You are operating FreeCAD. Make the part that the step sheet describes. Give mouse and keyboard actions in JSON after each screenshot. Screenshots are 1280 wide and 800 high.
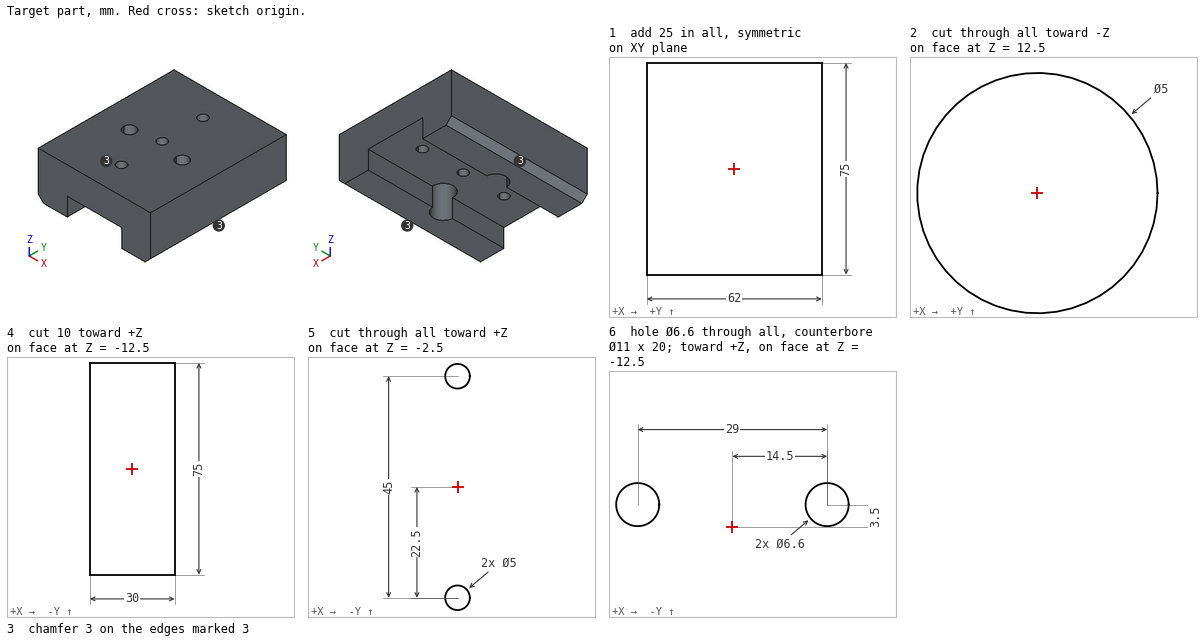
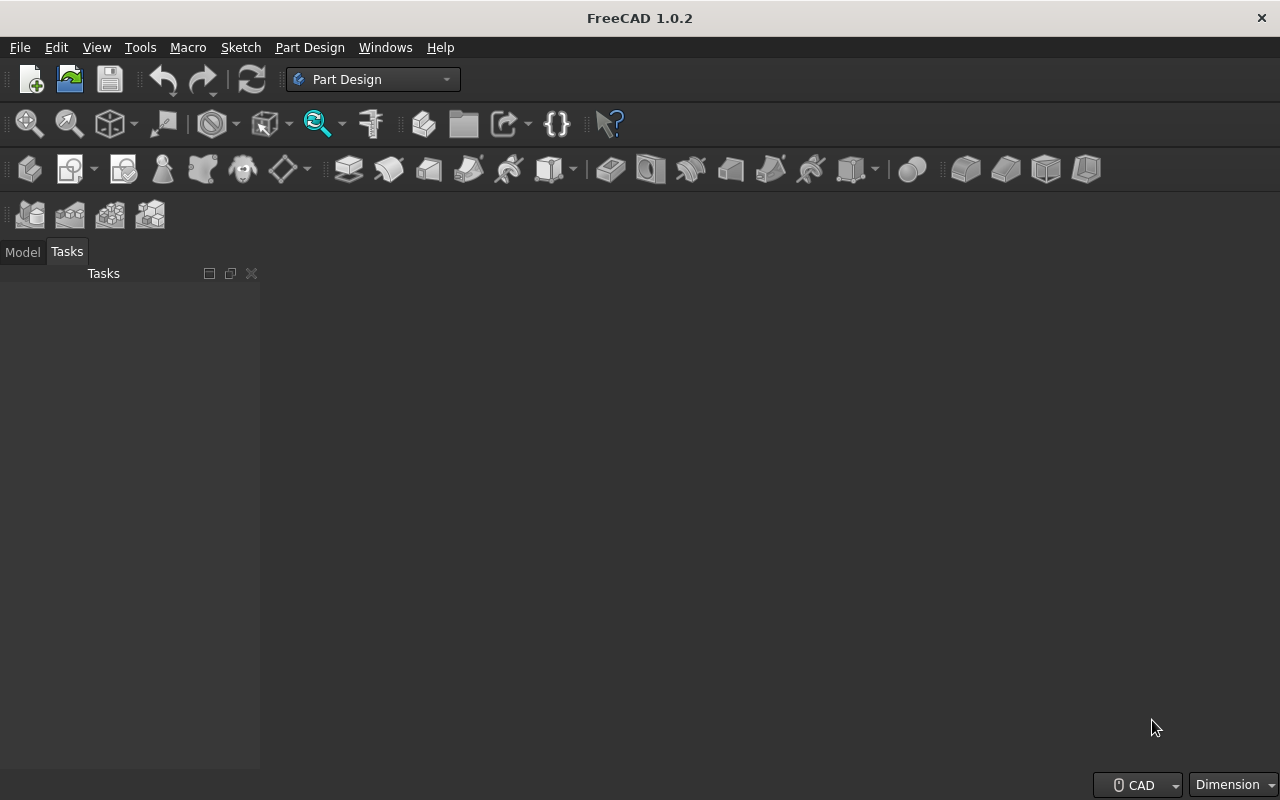
{"action": "left_click", "coordinate": [30, 80]}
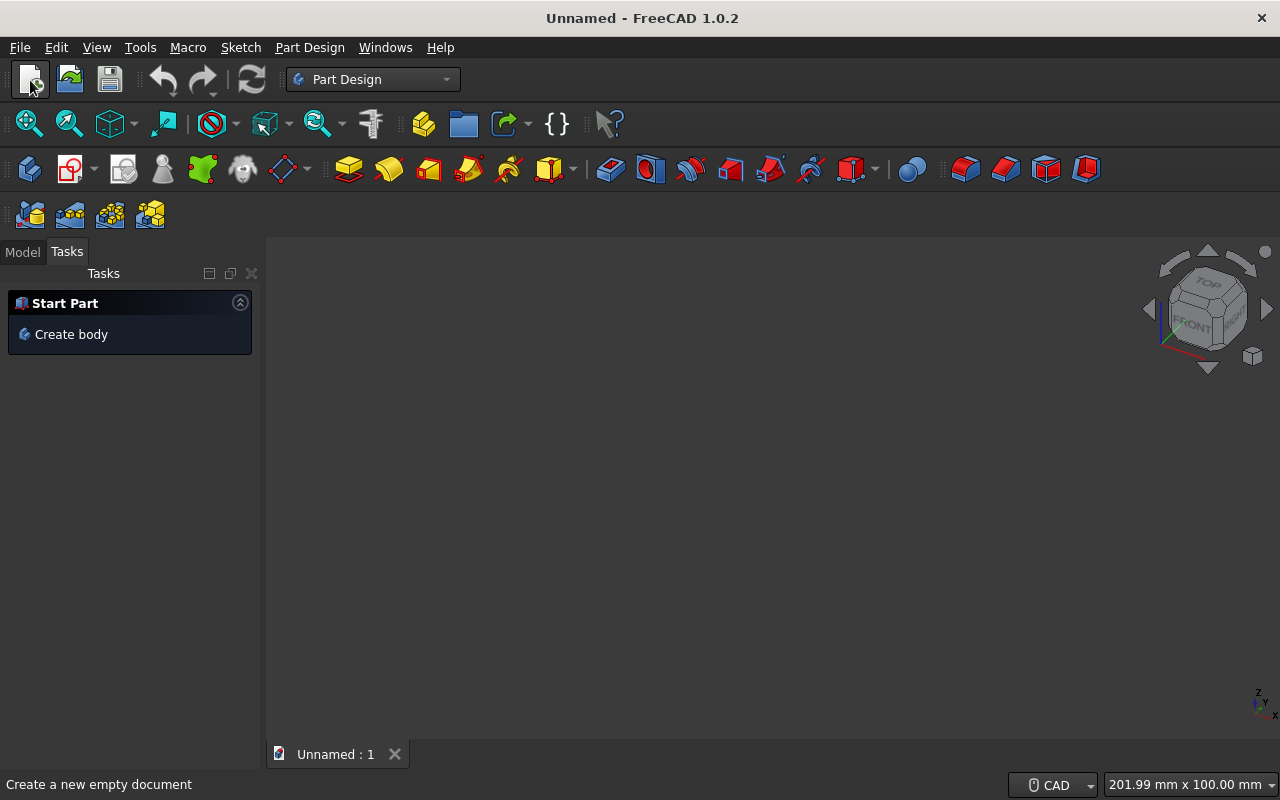
{"action": "left_click", "coordinate": [70, 170]}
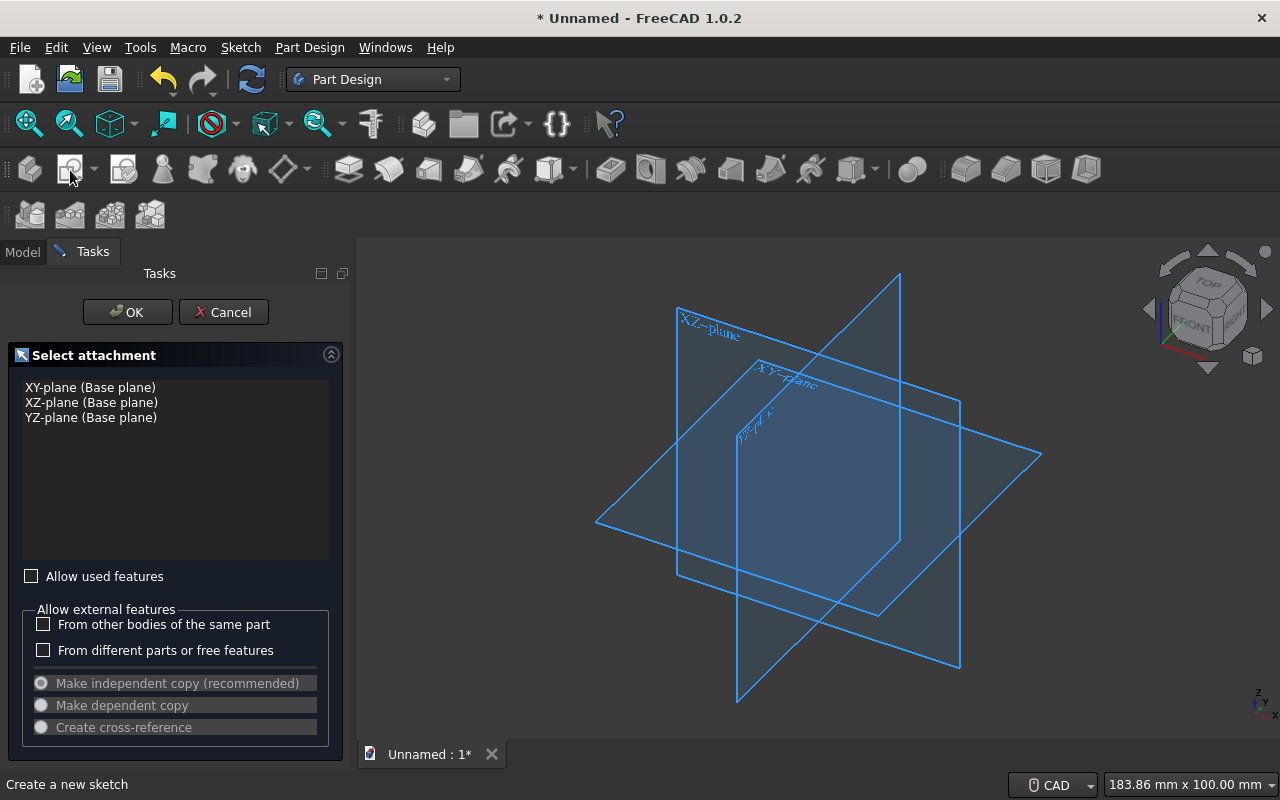
{"action": "left_click", "coordinate": [82, 388]}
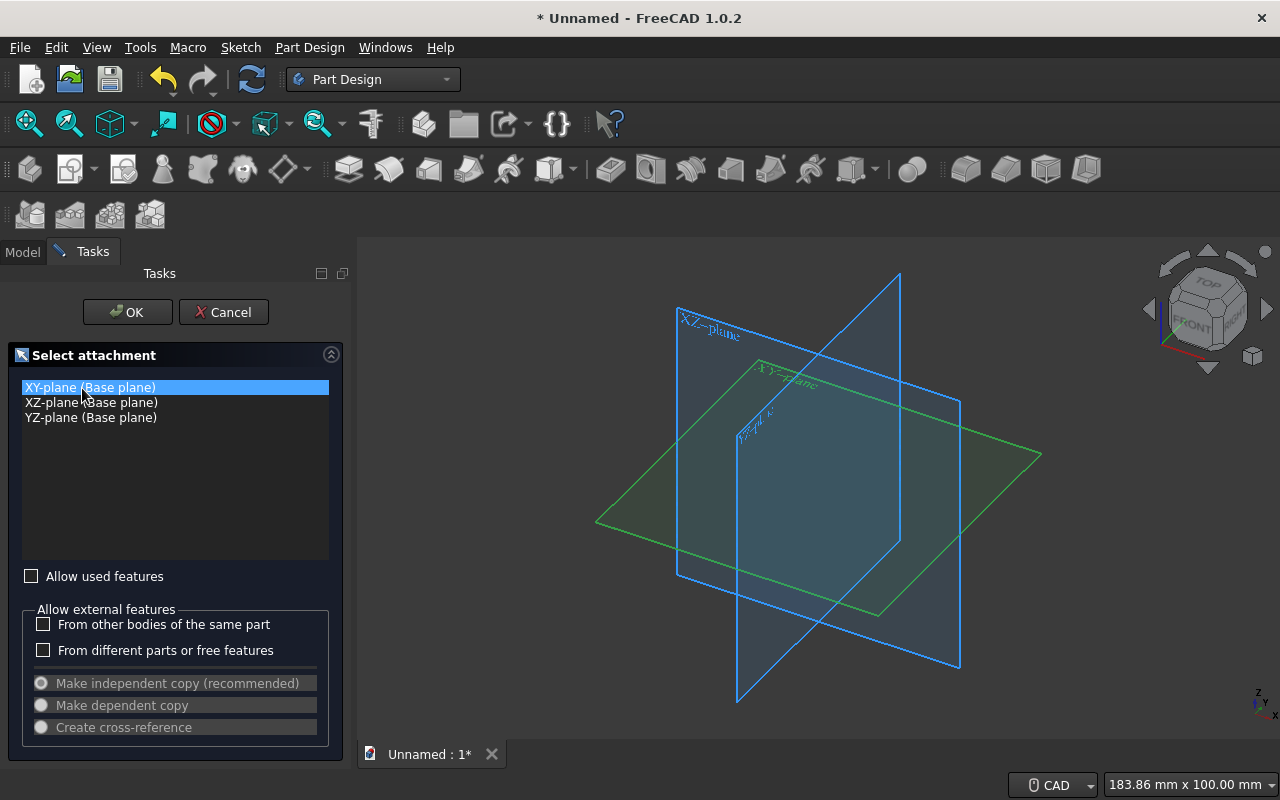
{"action": "left_click", "coordinate": [128, 312]}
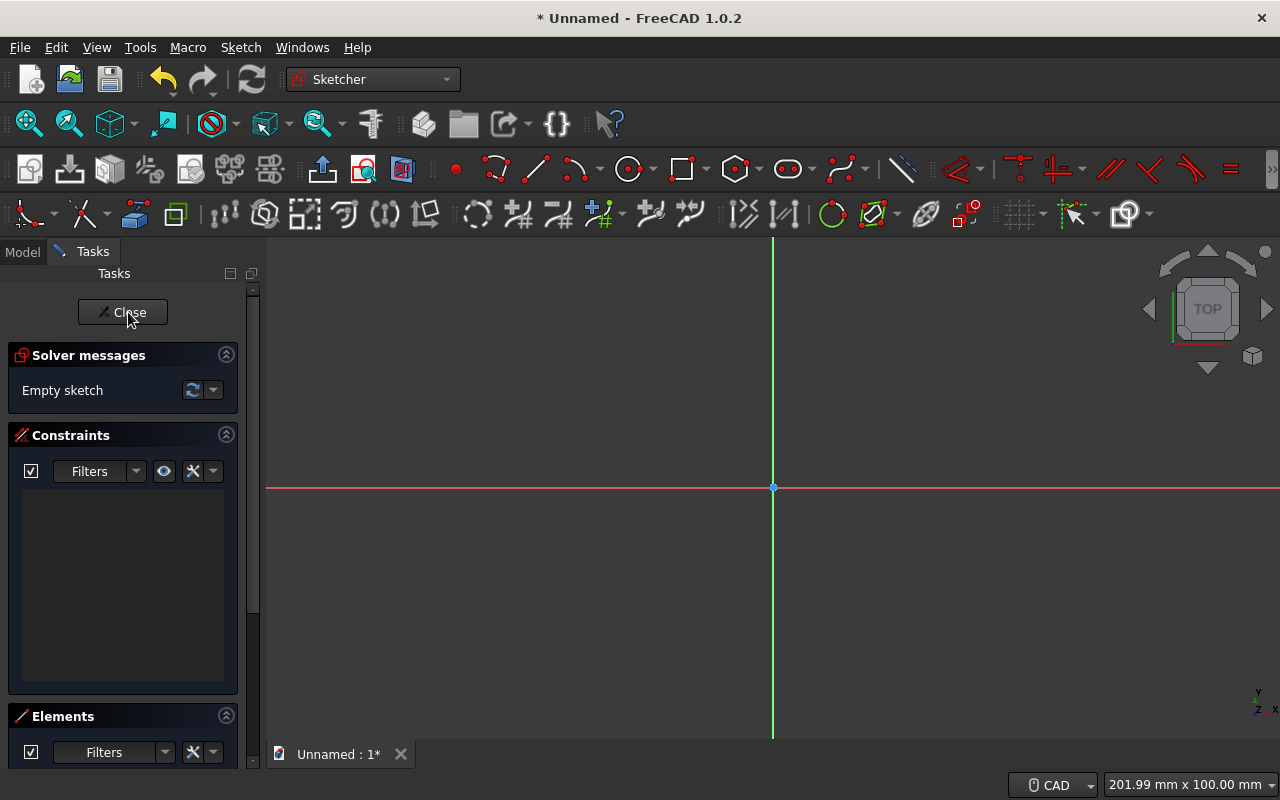
{"action": "key", "text": "g v"}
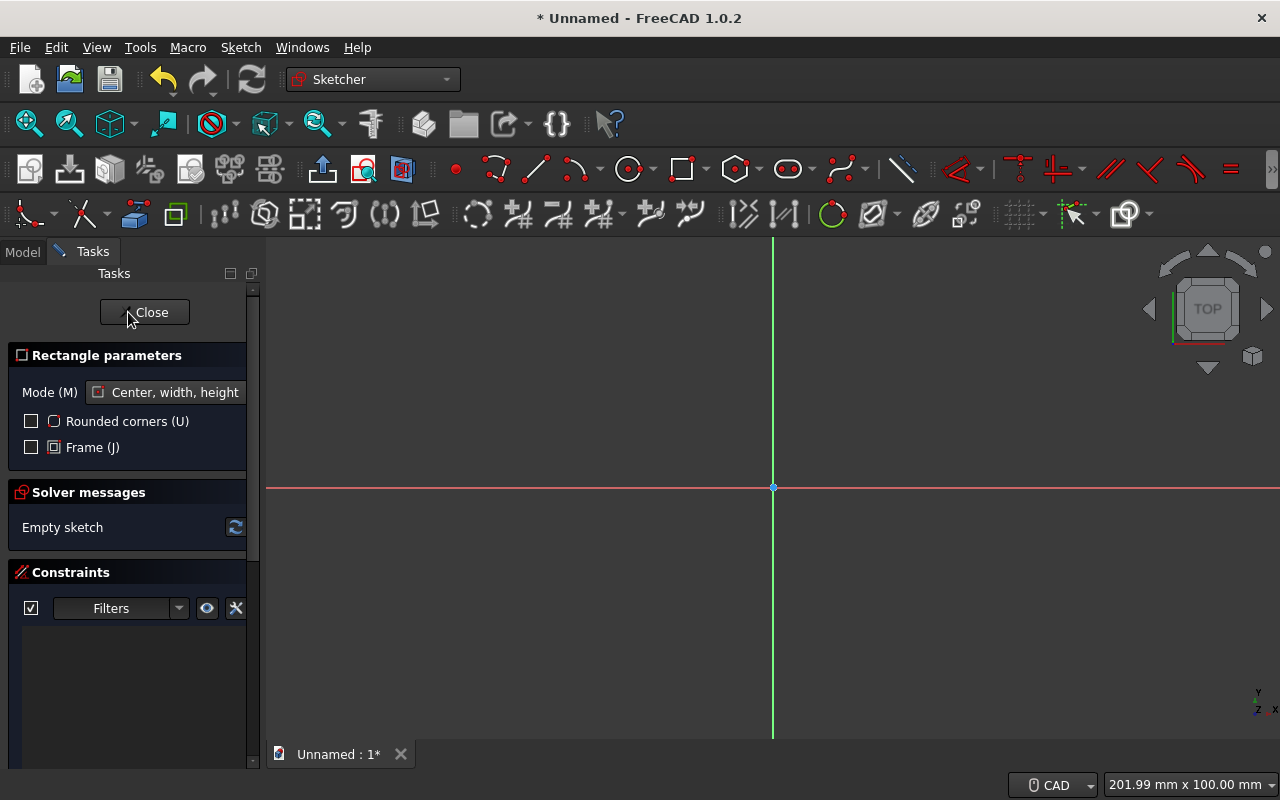
{"action": "left_click", "coordinate": [773, 488]}
{"action": "left_click", "coordinate": [929, 300]}
{"action": "key", "text": "Escape"}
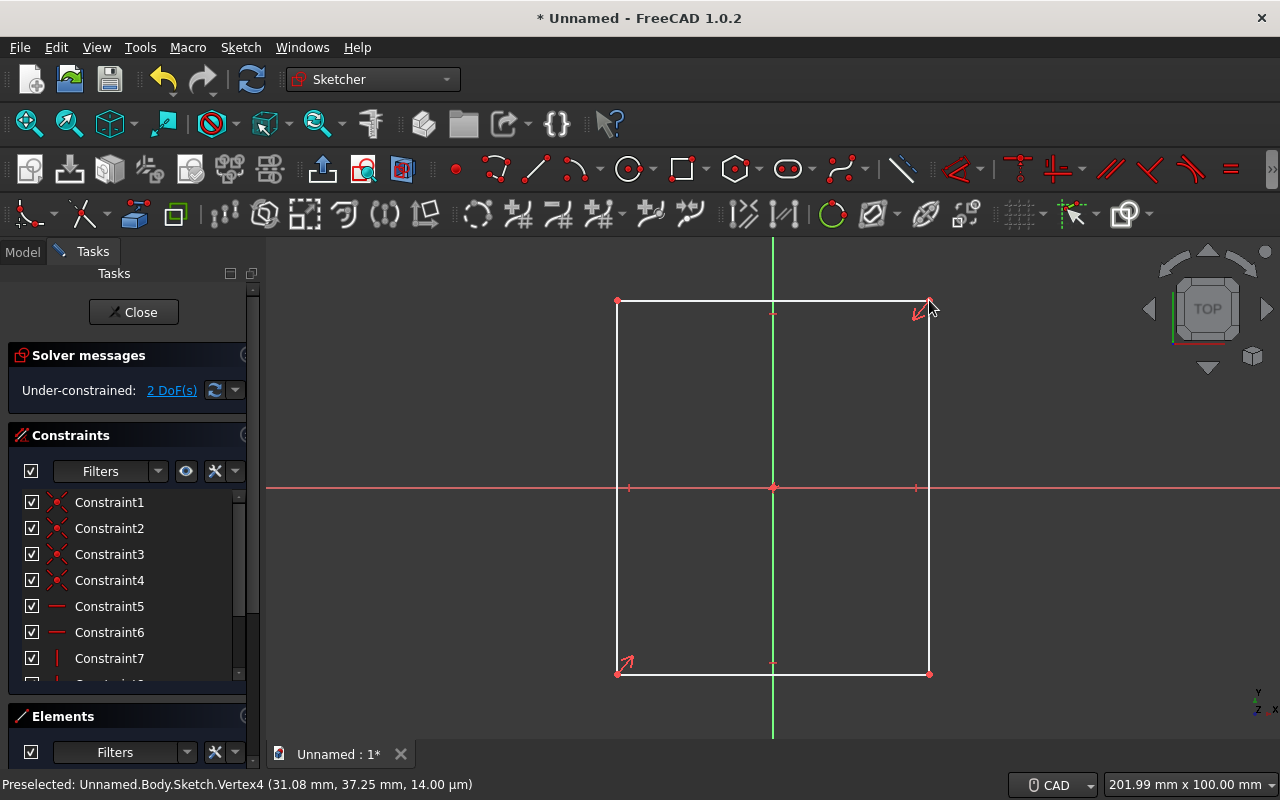
{"action": "key", "text": "d"}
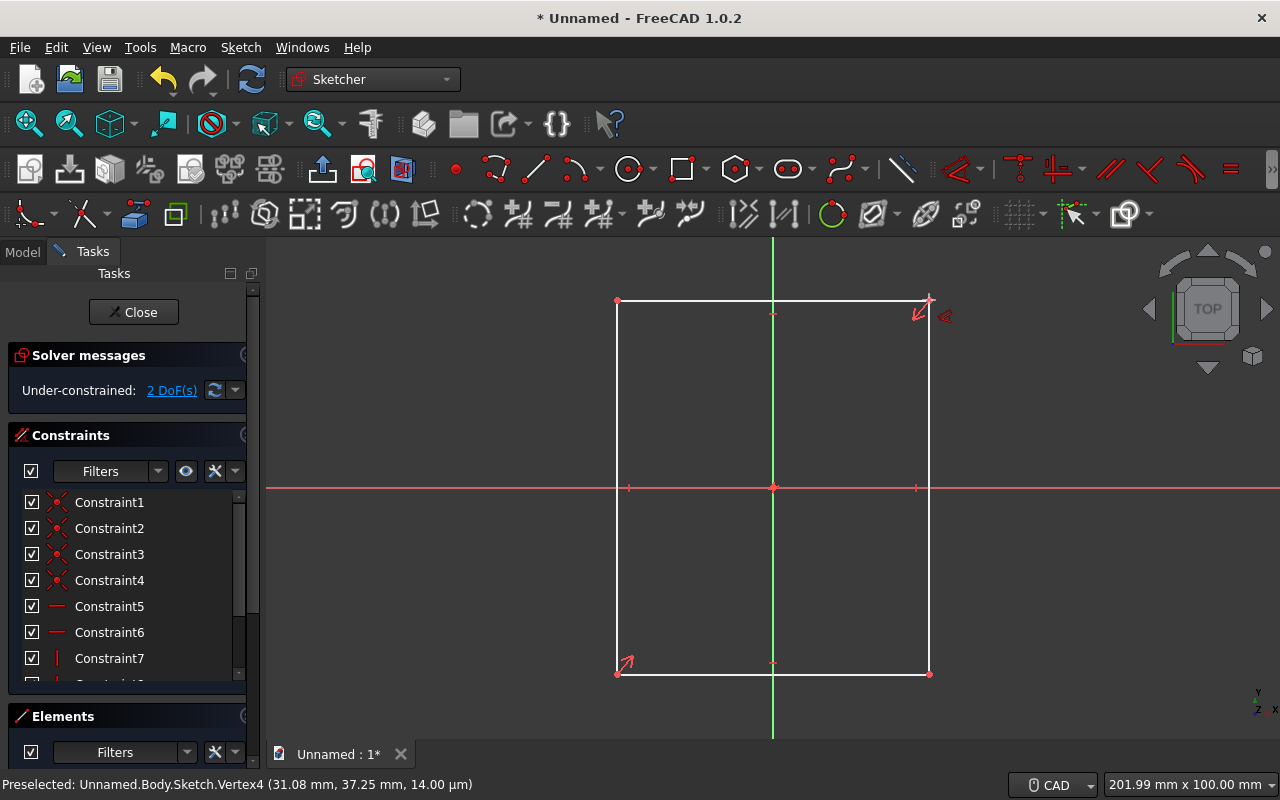
{"action": "left_click", "coordinate": [711, 675]}
{"action": "left_click", "coordinate": [701, 709]}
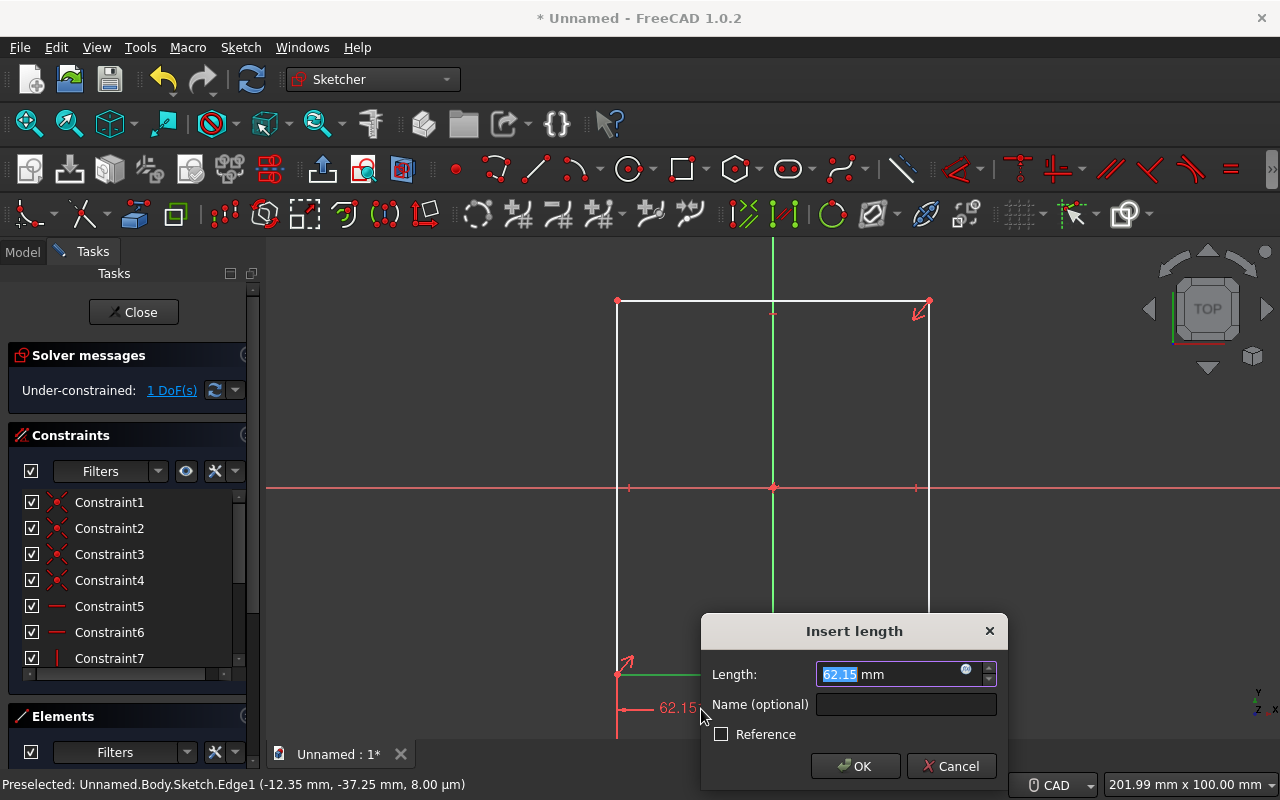
{"action": "type", "text": "62"}
{"action": "key", "text": "Return"}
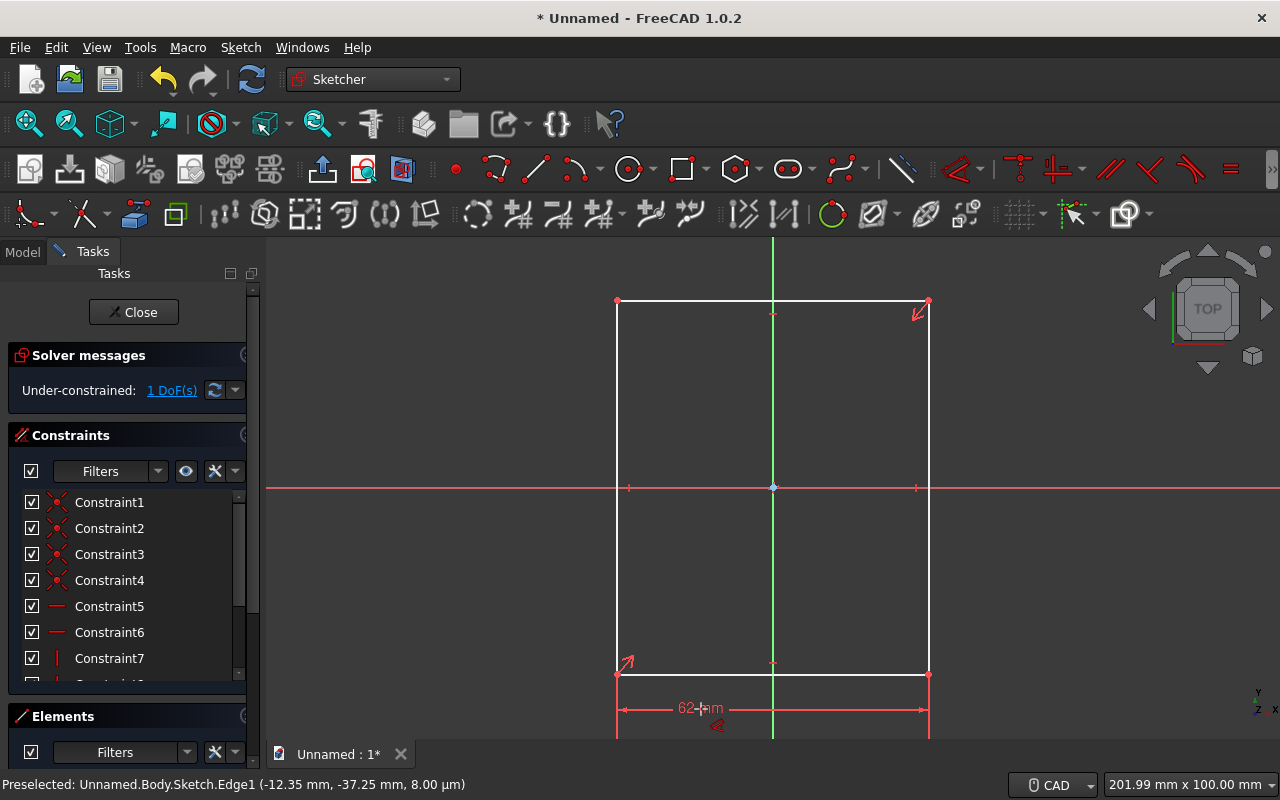
{"action": "left_click", "coordinate": [929, 563]}
{"action": "left_click", "coordinate": [963, 402]}